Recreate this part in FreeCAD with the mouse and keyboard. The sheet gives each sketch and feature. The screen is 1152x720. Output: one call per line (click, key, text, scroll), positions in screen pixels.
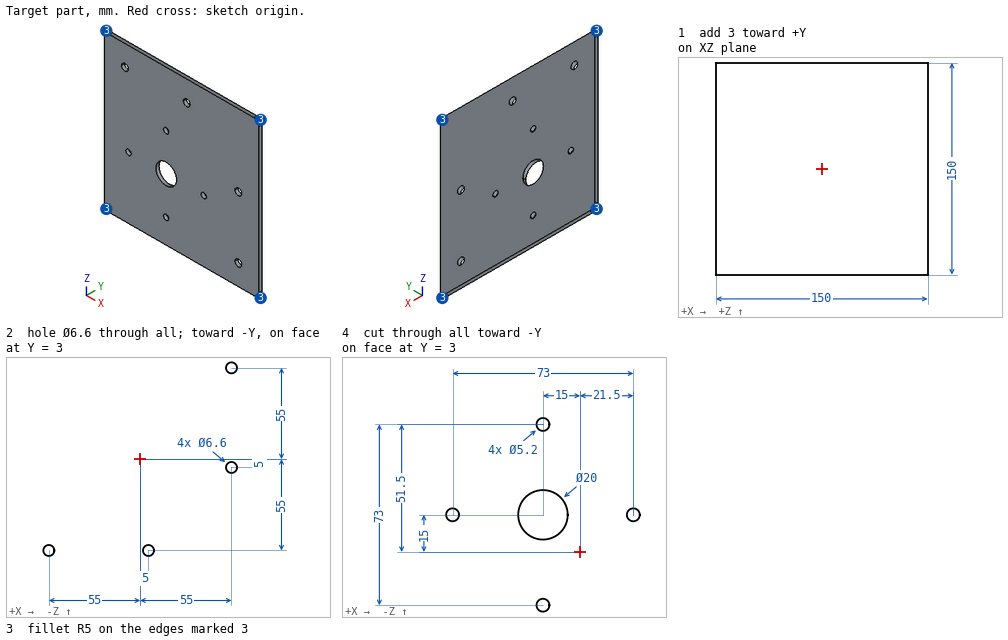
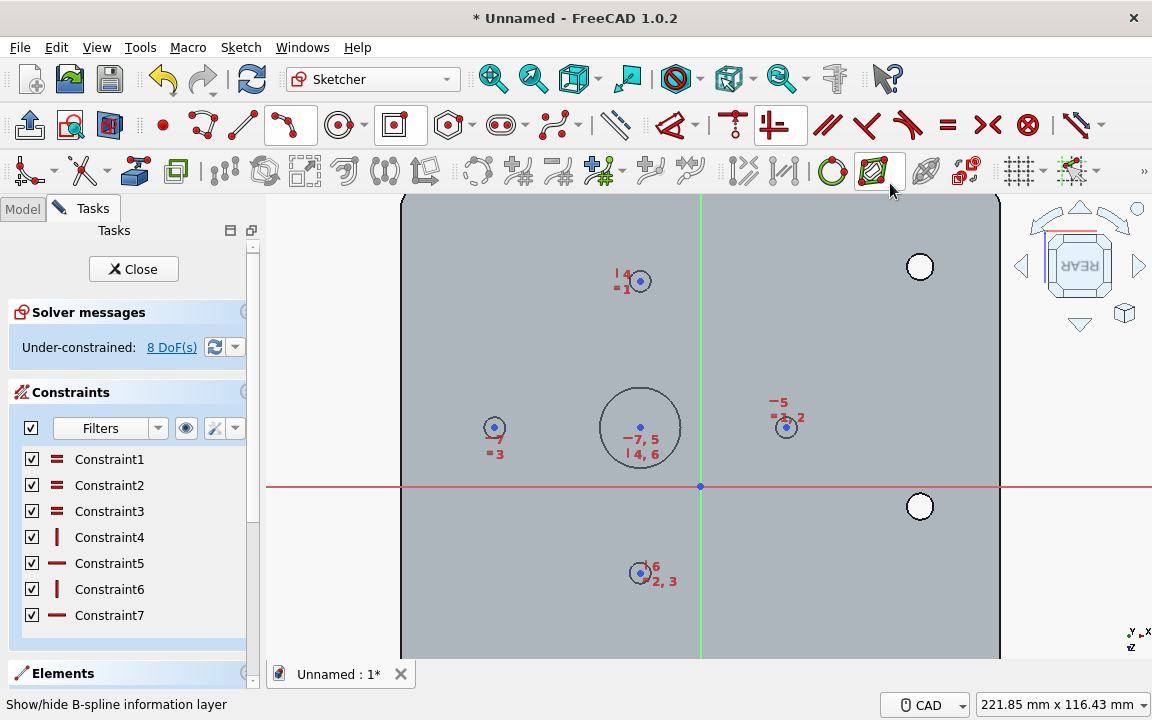
click(670, 126)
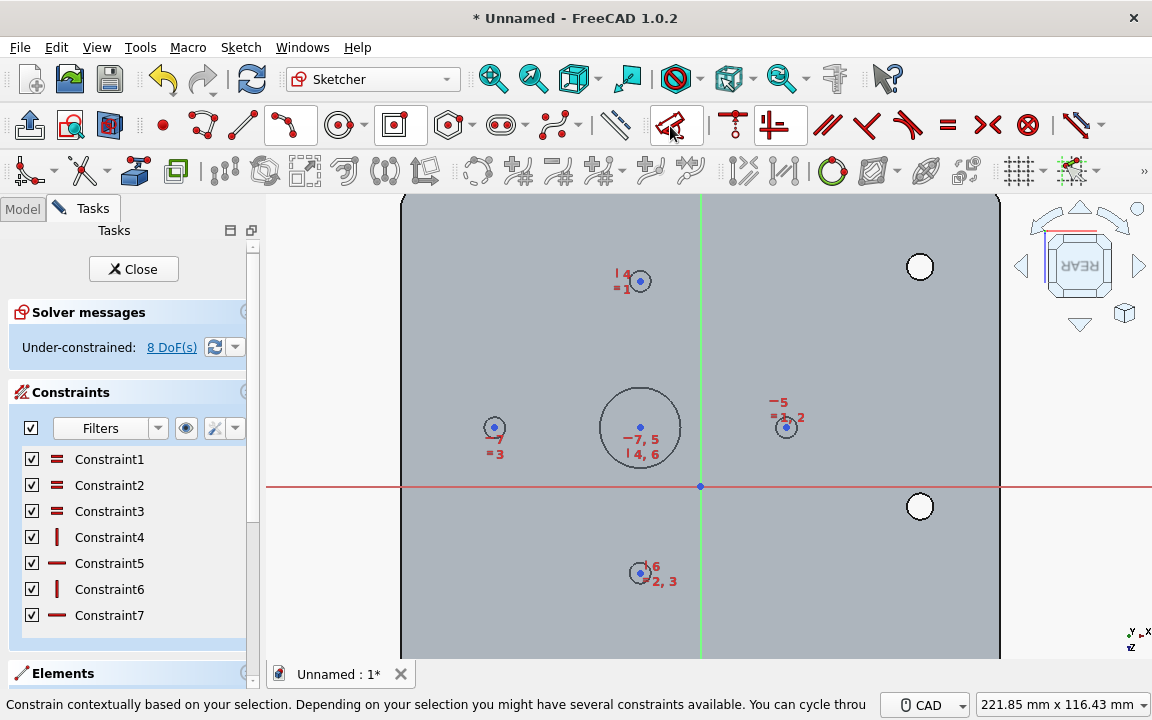
click(669, 399)
click(661, 358)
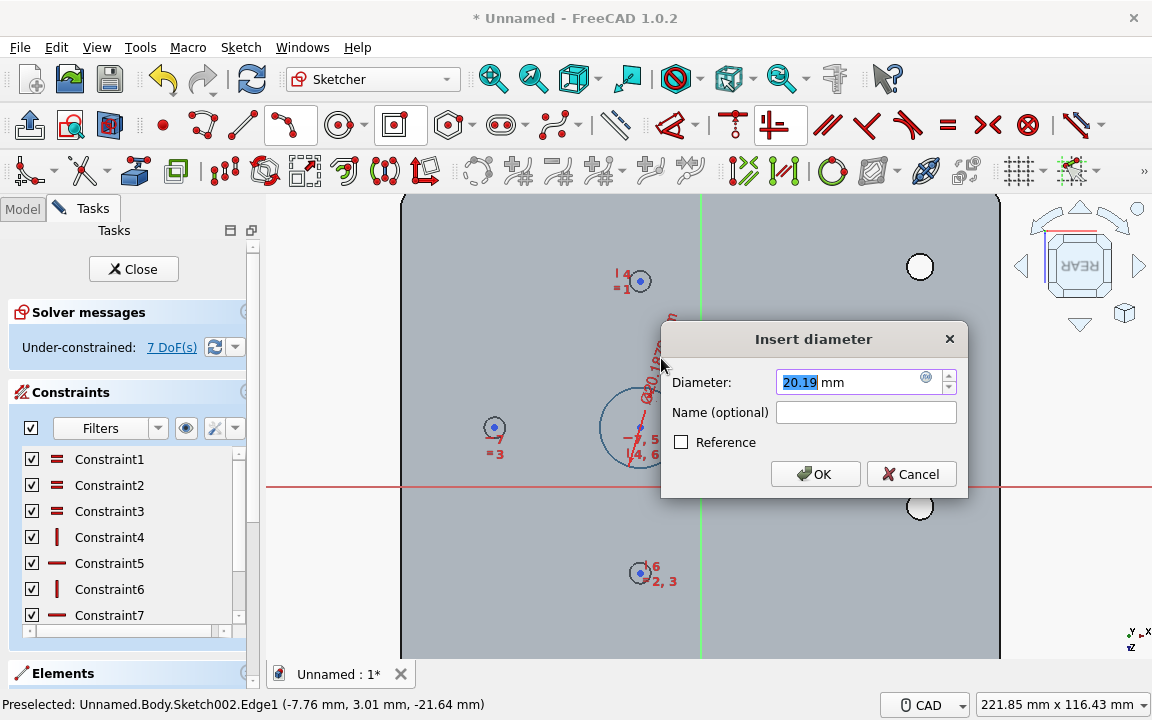
text(20)
key(Return)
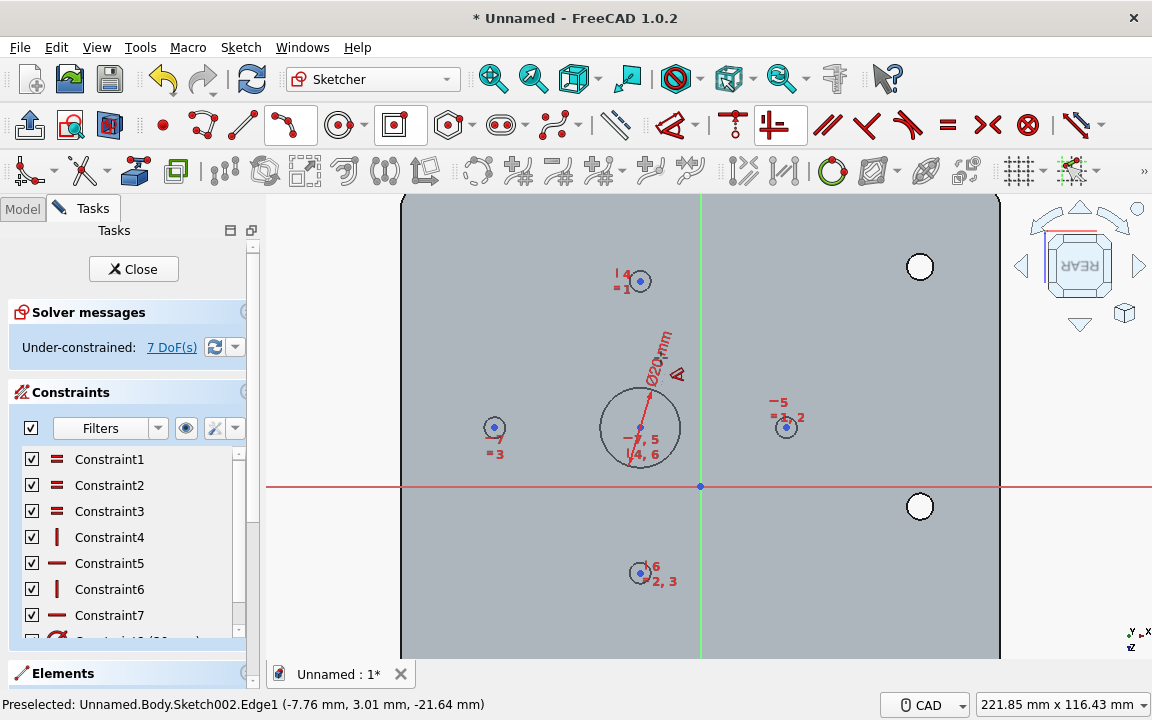
scroll(648, 274, up, 4)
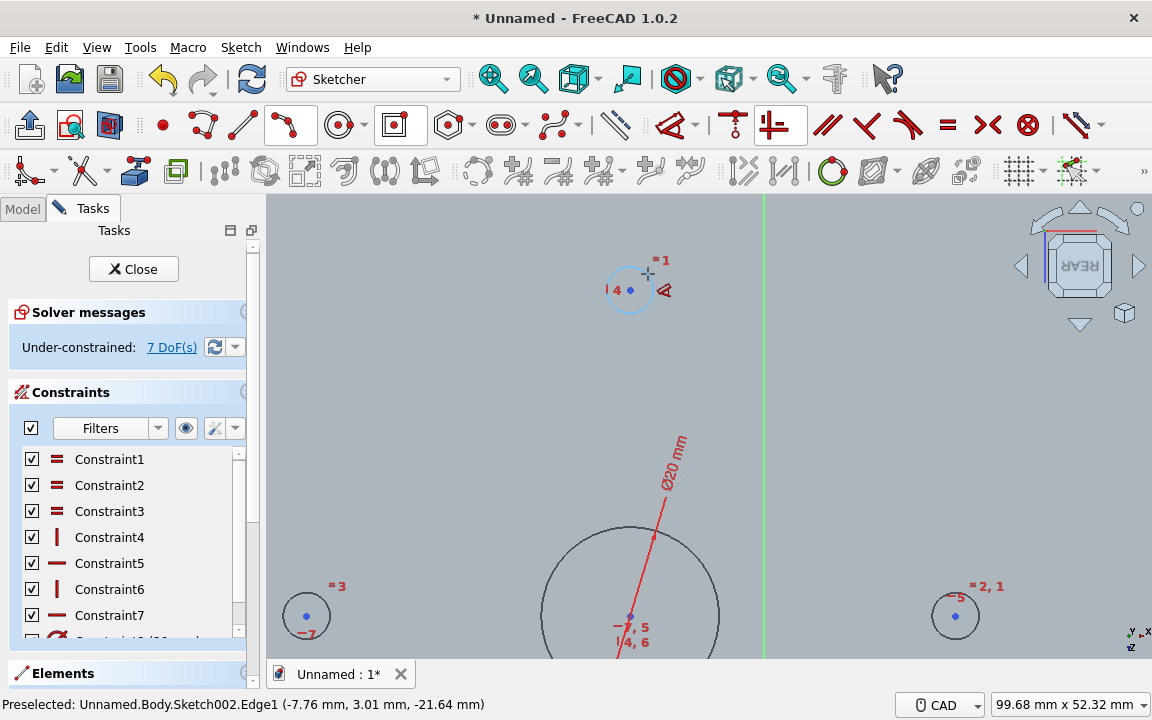
click(647, 274)
click(670, 252)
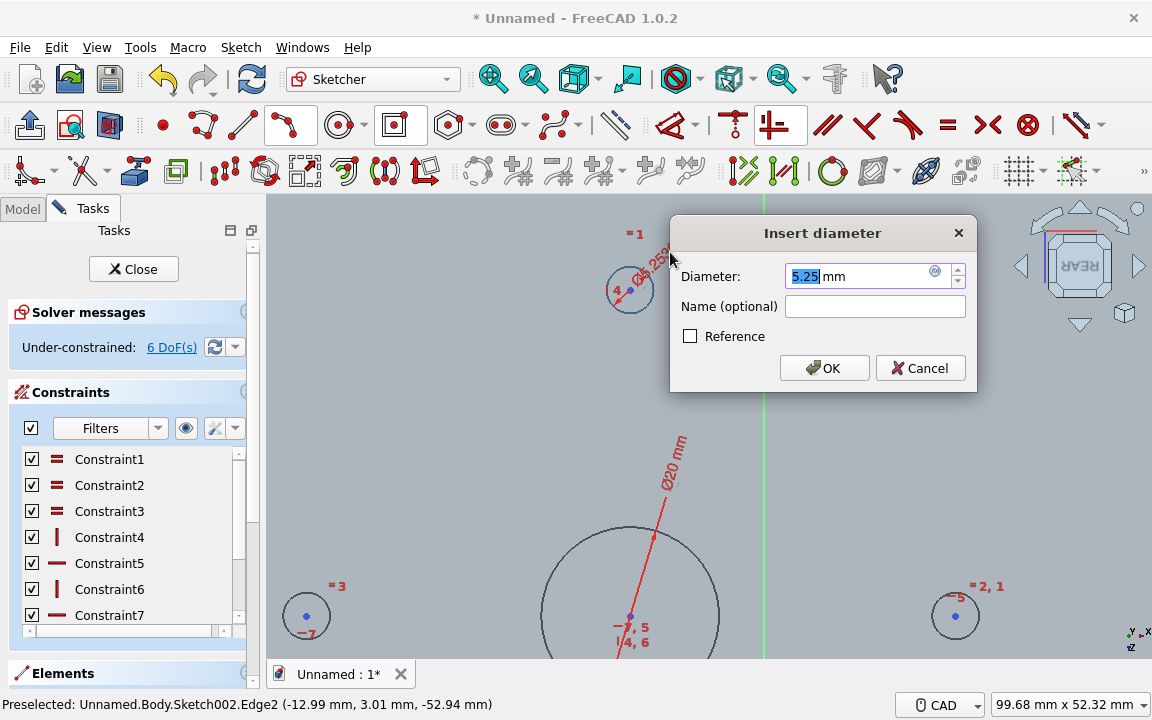
text(5.2)
key(Return)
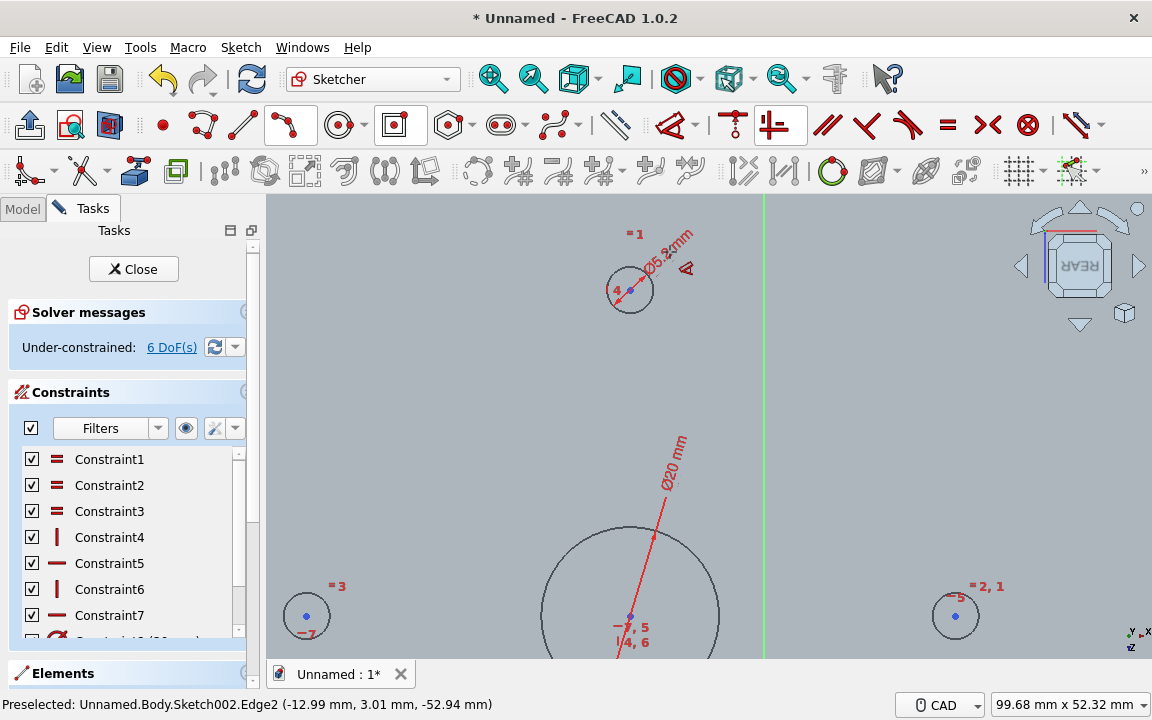
click(630, 616)
click(697, 582)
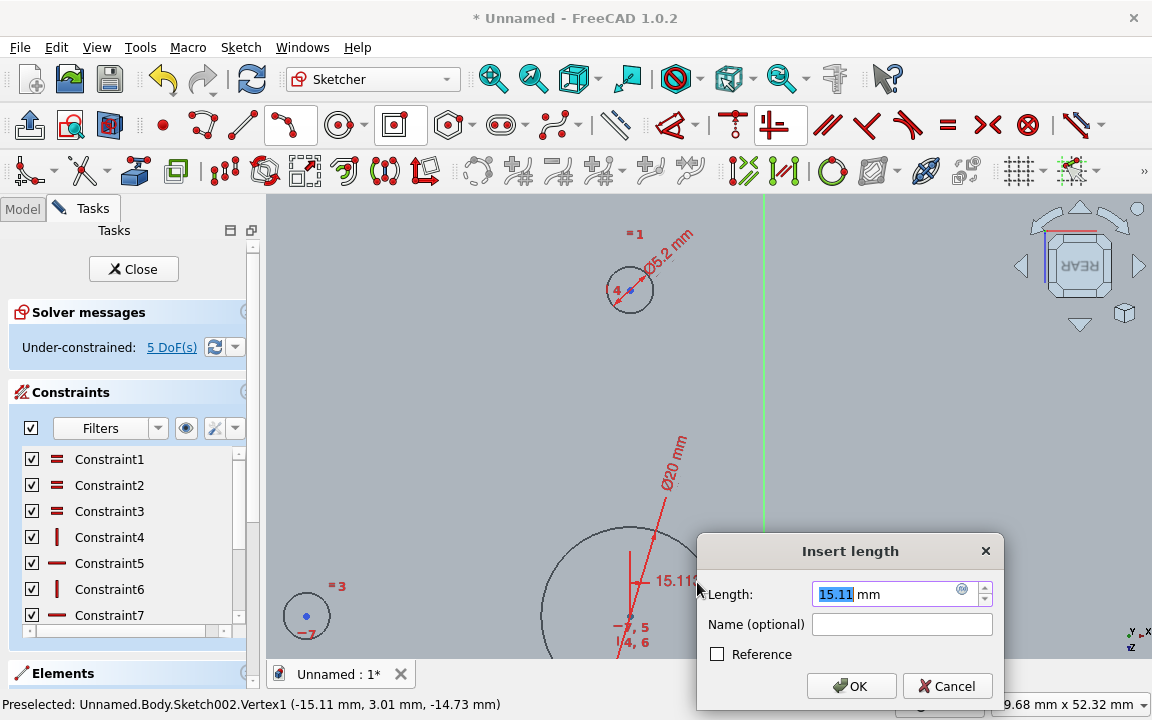
text(15)
key(Return)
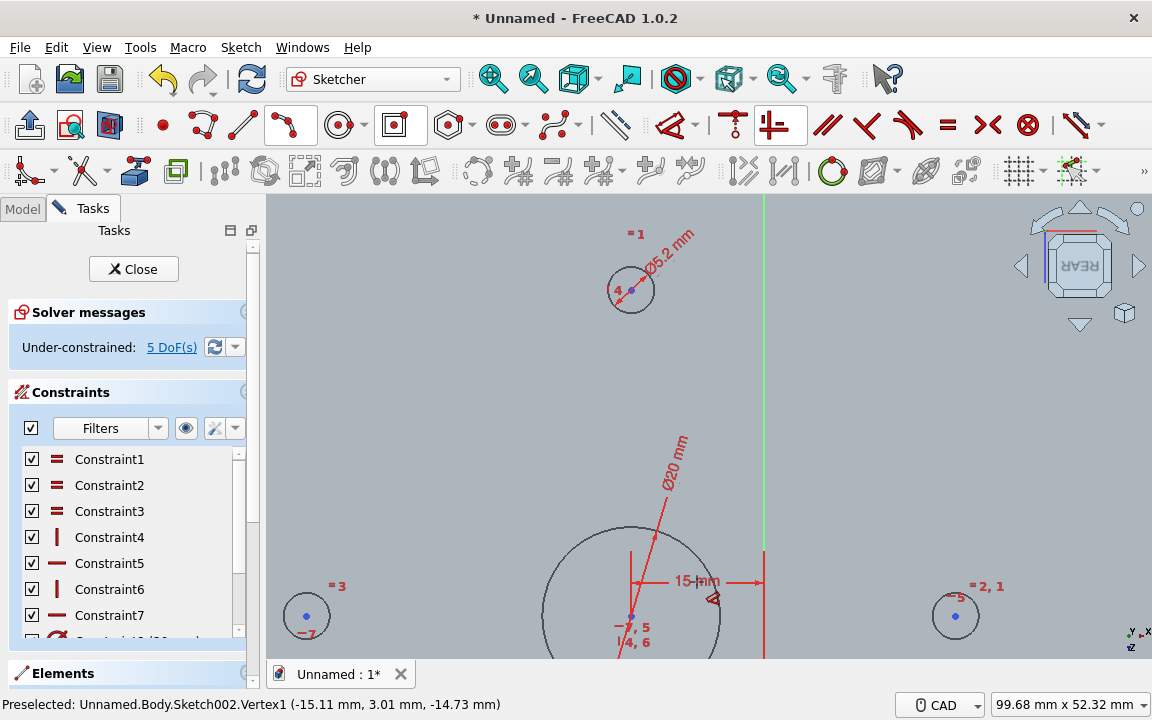
click(631, 616)
click(798, 624)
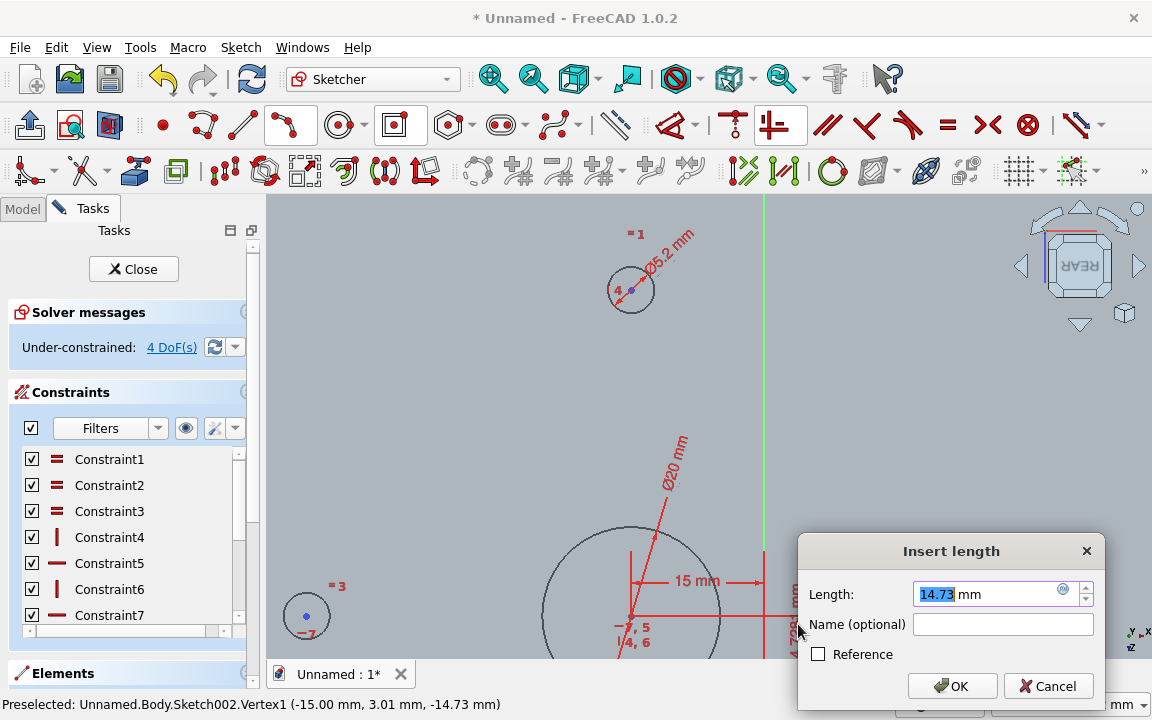
text(15)
key(Return)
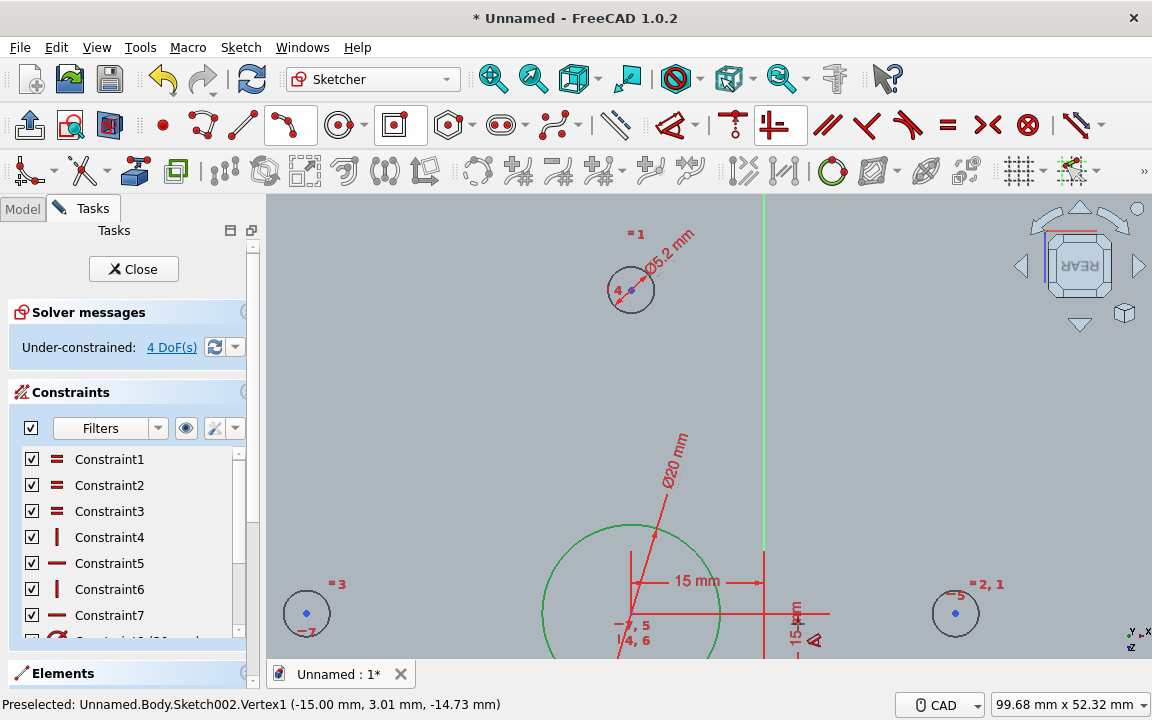
click(631, 290)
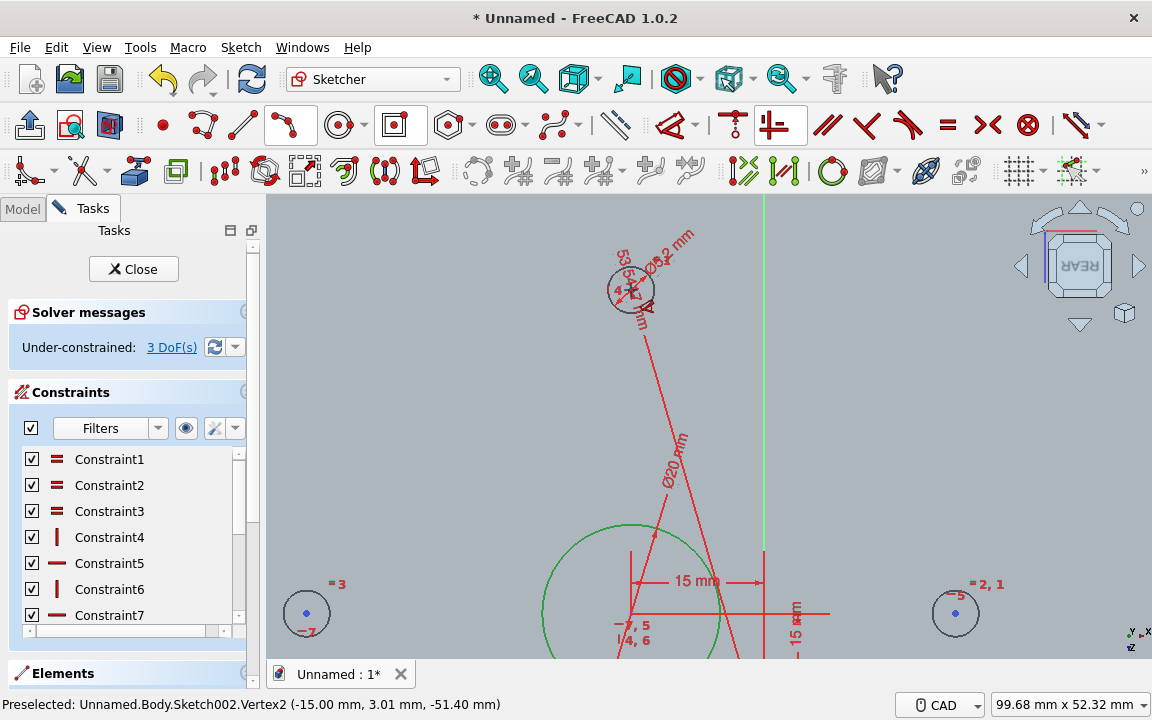
scroll(648, 274, down, 4)